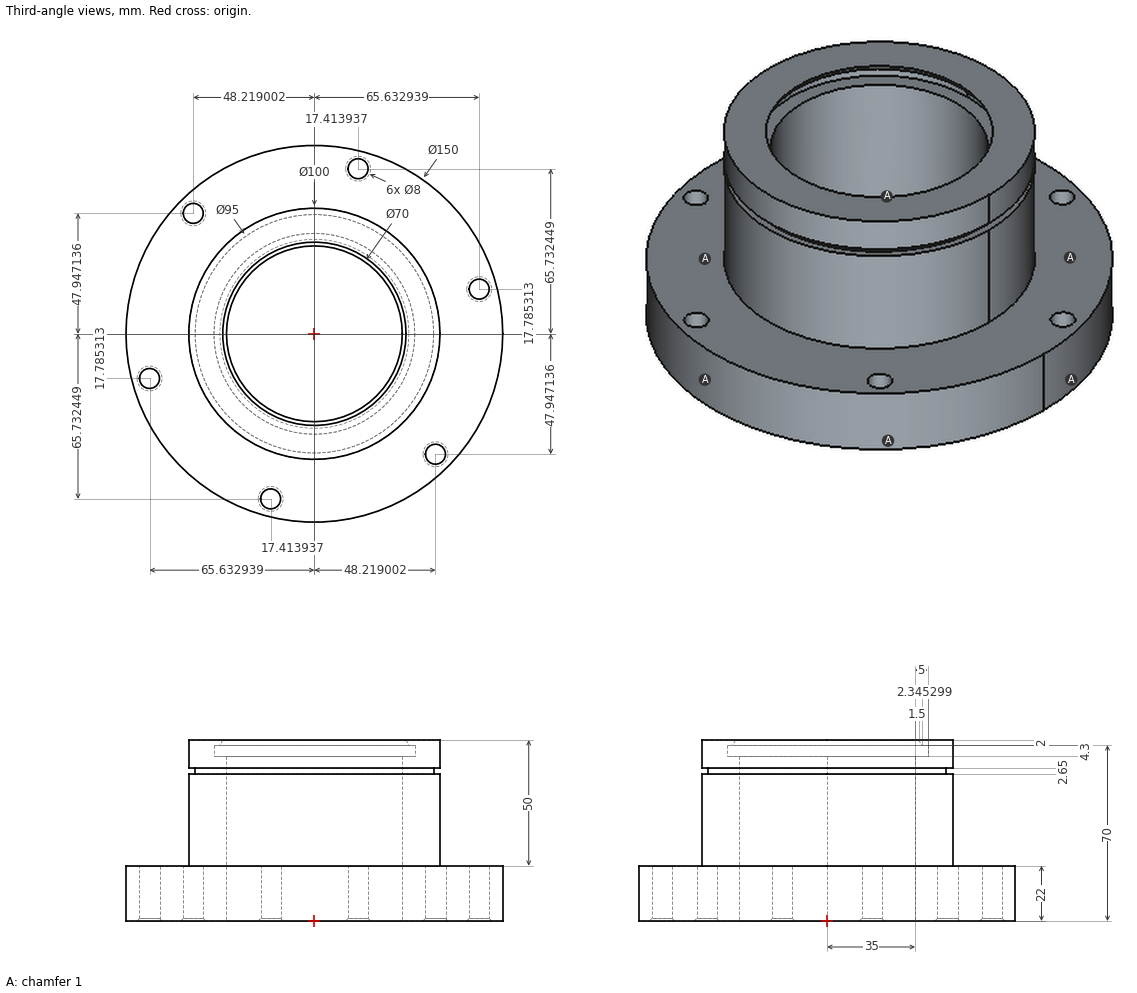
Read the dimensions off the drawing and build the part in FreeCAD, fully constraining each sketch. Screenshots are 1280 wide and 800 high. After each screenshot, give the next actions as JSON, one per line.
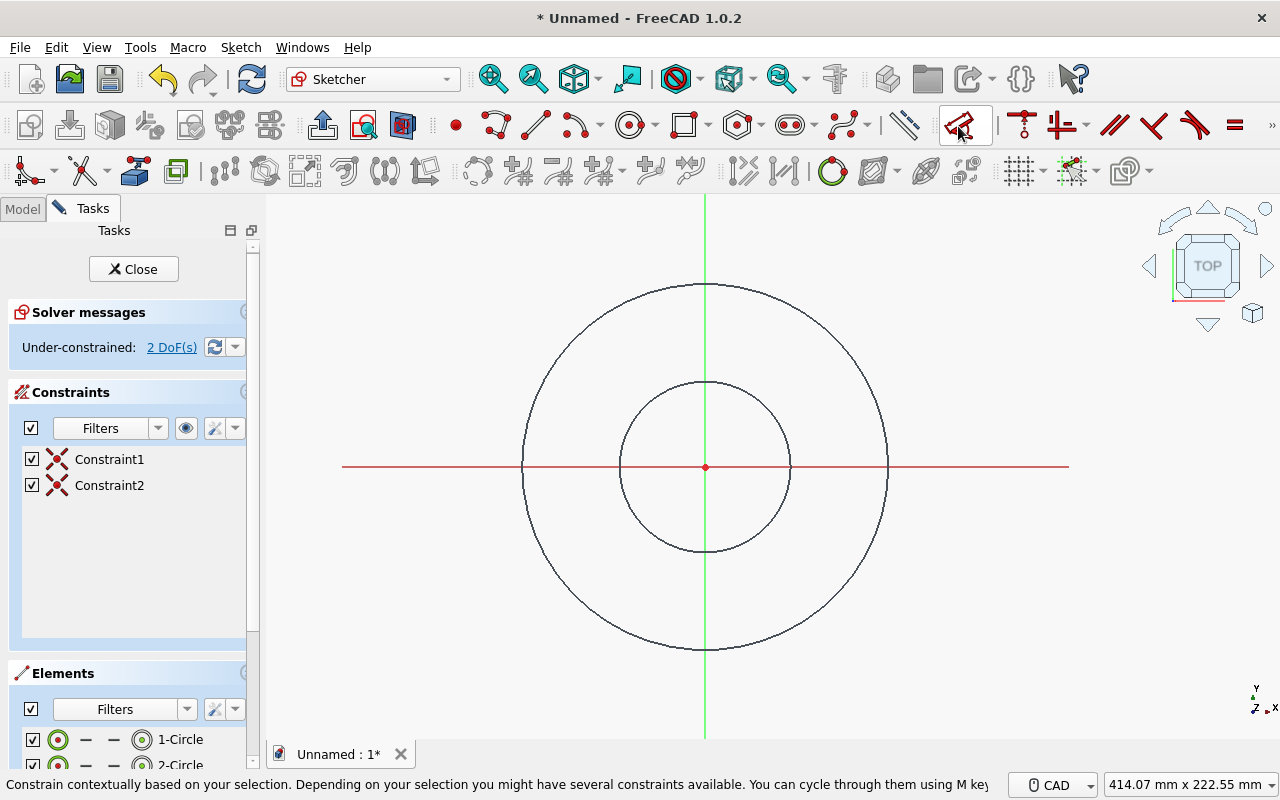
{"action": "left_click", "coordinate": [834, 337]}
{"action": "left_click", "coordinate": [857, 314]}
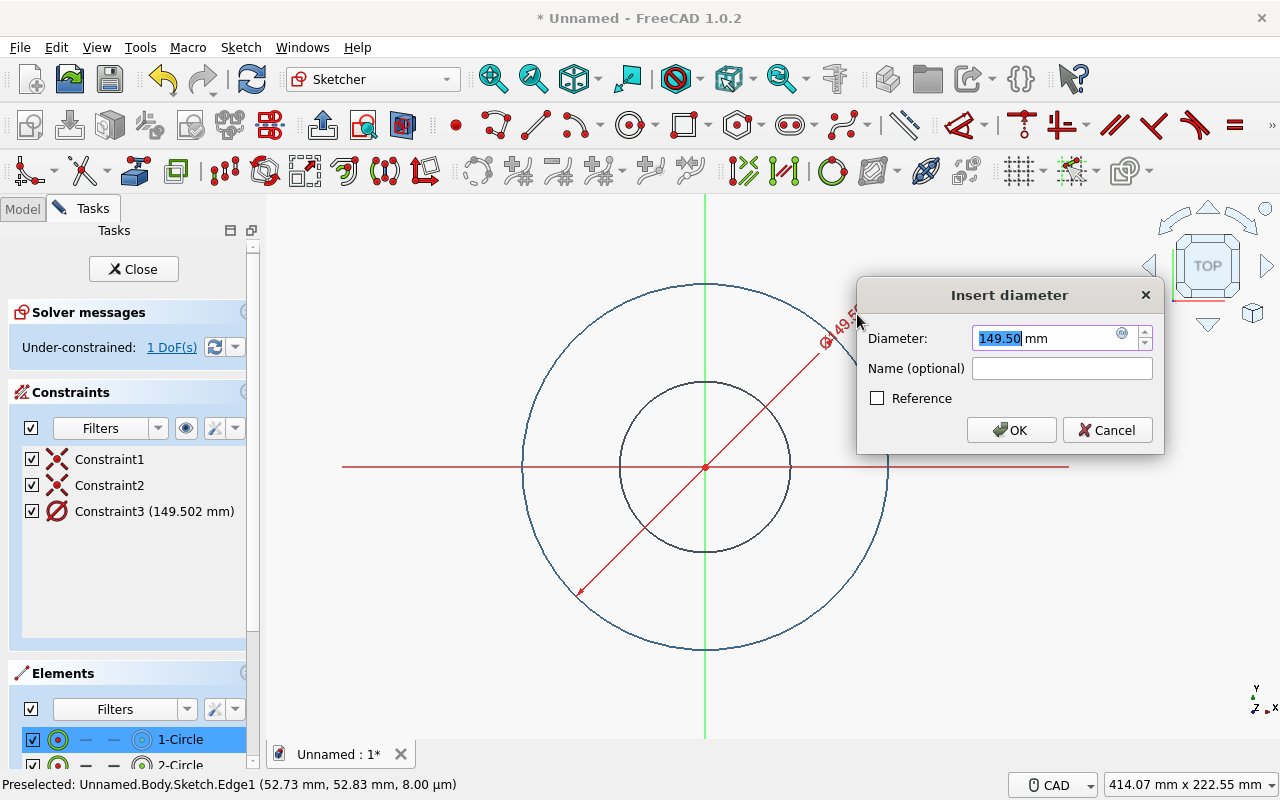
{"action": "type", "text": "150"}
{"action": "key", "text": "Return"}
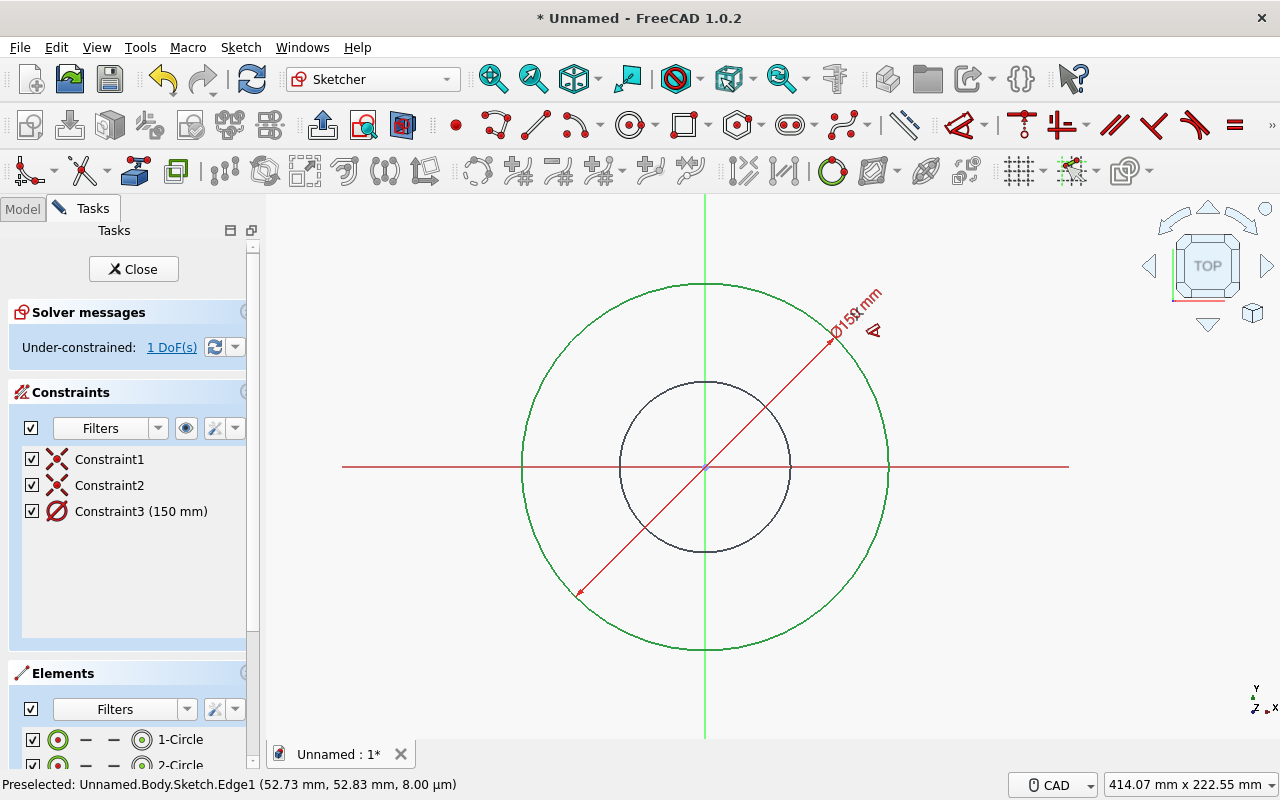
{"action": "left_click", "coordinate": [765, 406]}
{"action": "left_click", "coordinate": [787, 383]}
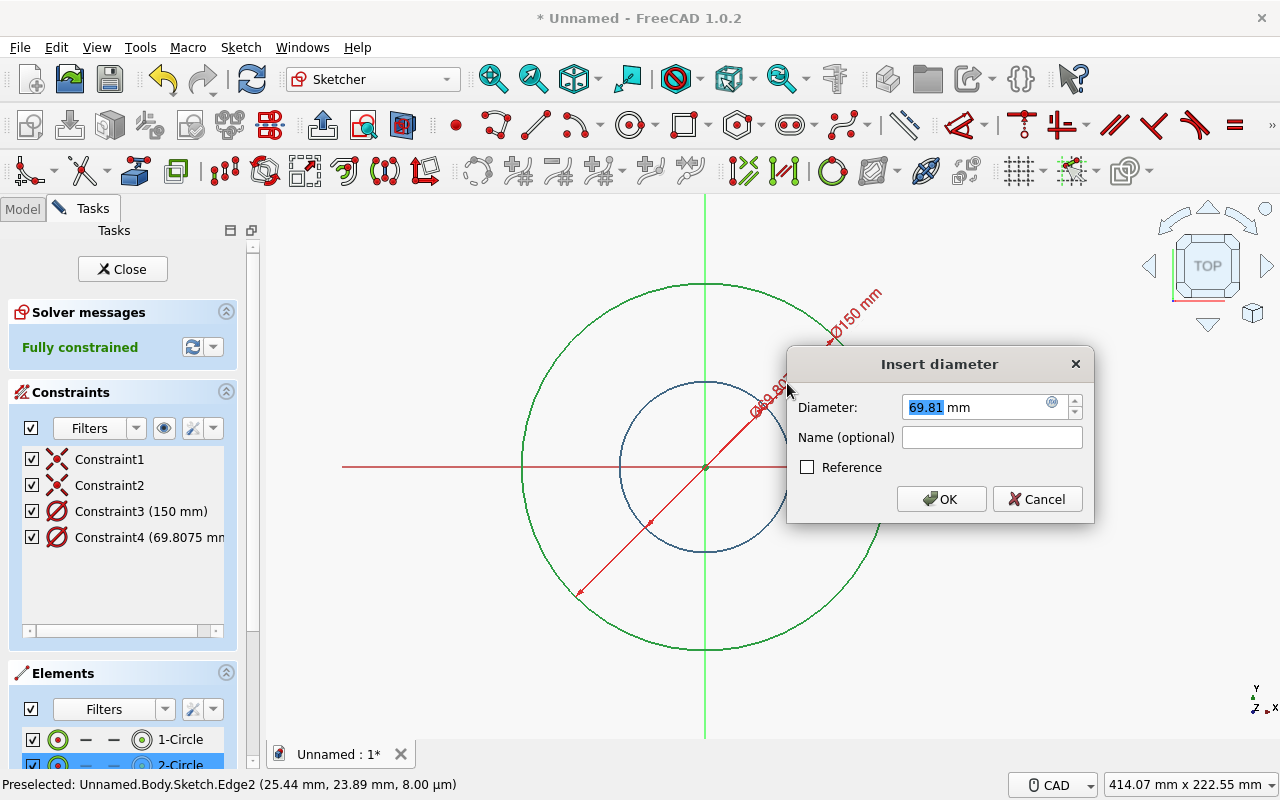
{"action": "type", "text": "70"}
{"action": "key", "text": "Return"}
{"action": "key", "text": "Escape"}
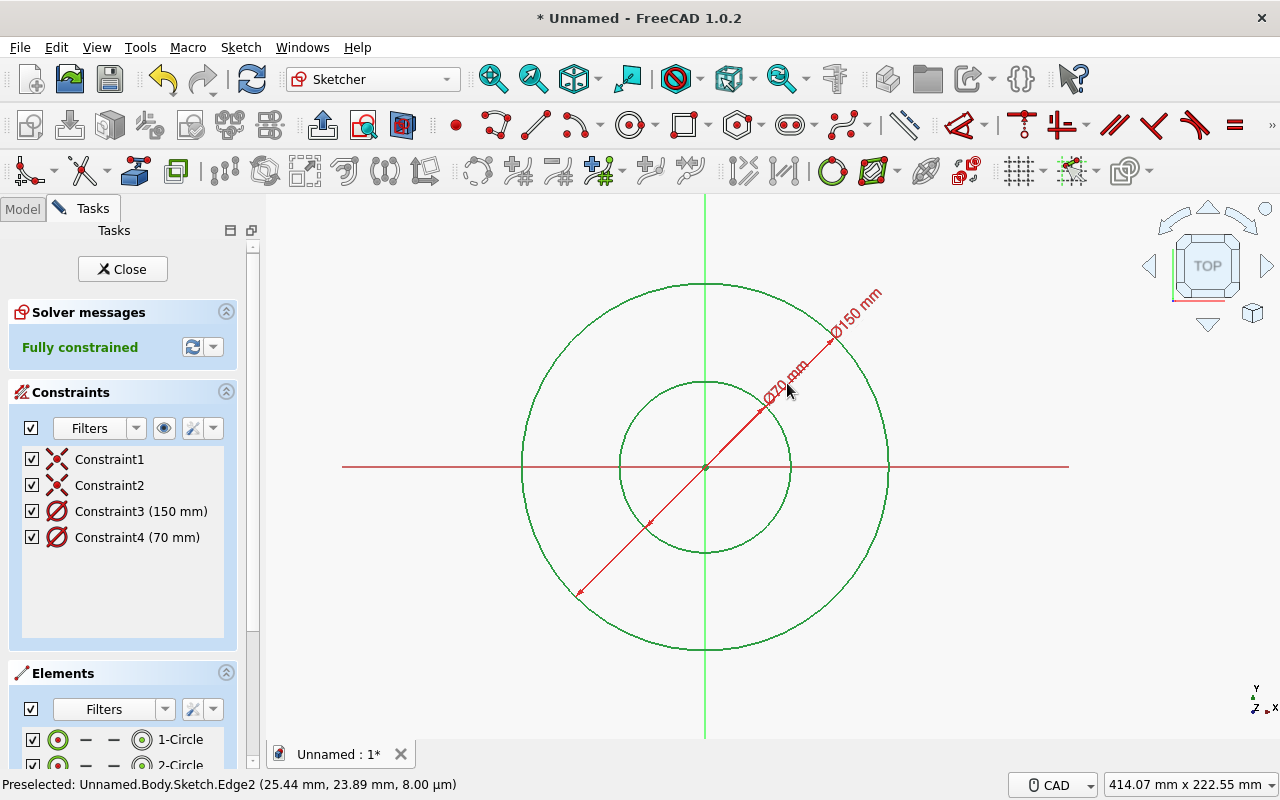
{"action": "left_click", "coordinate": [123, 269]}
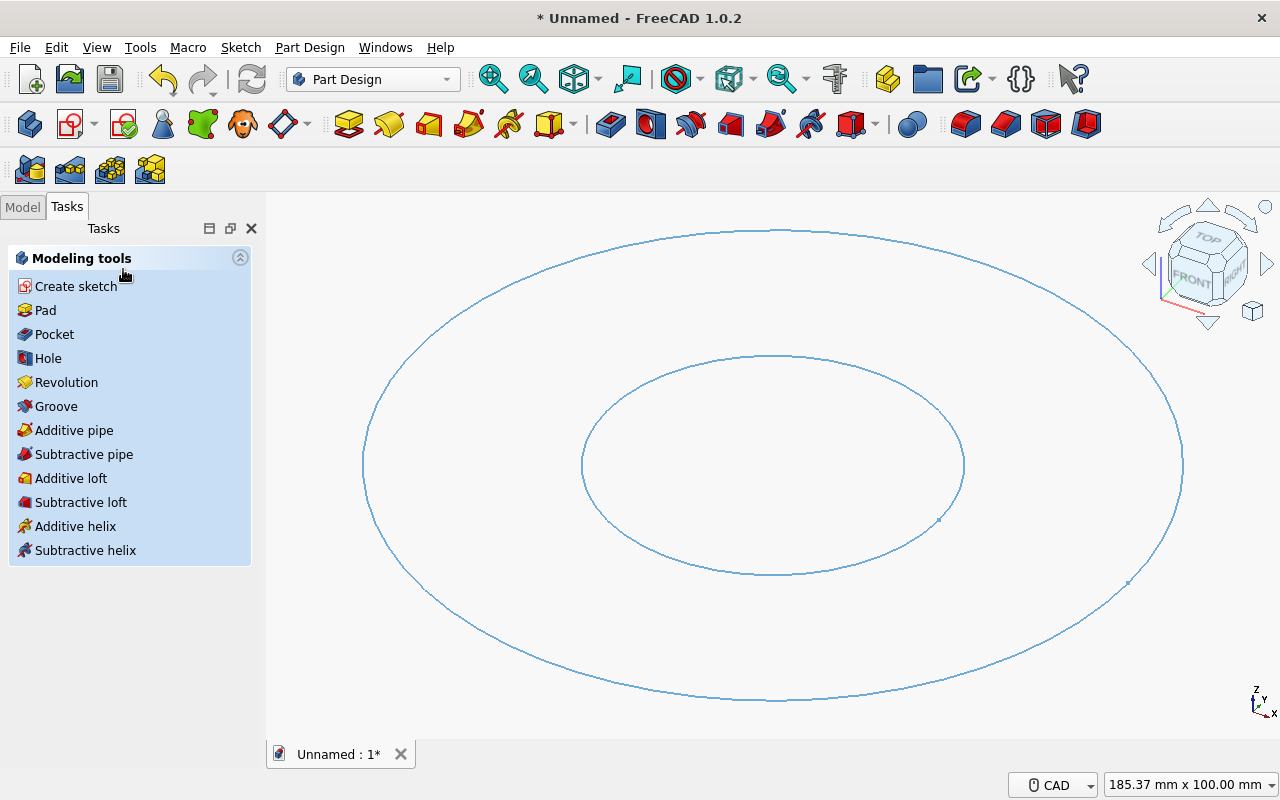
{"action": "left_click", "coordinate": [350, 124]}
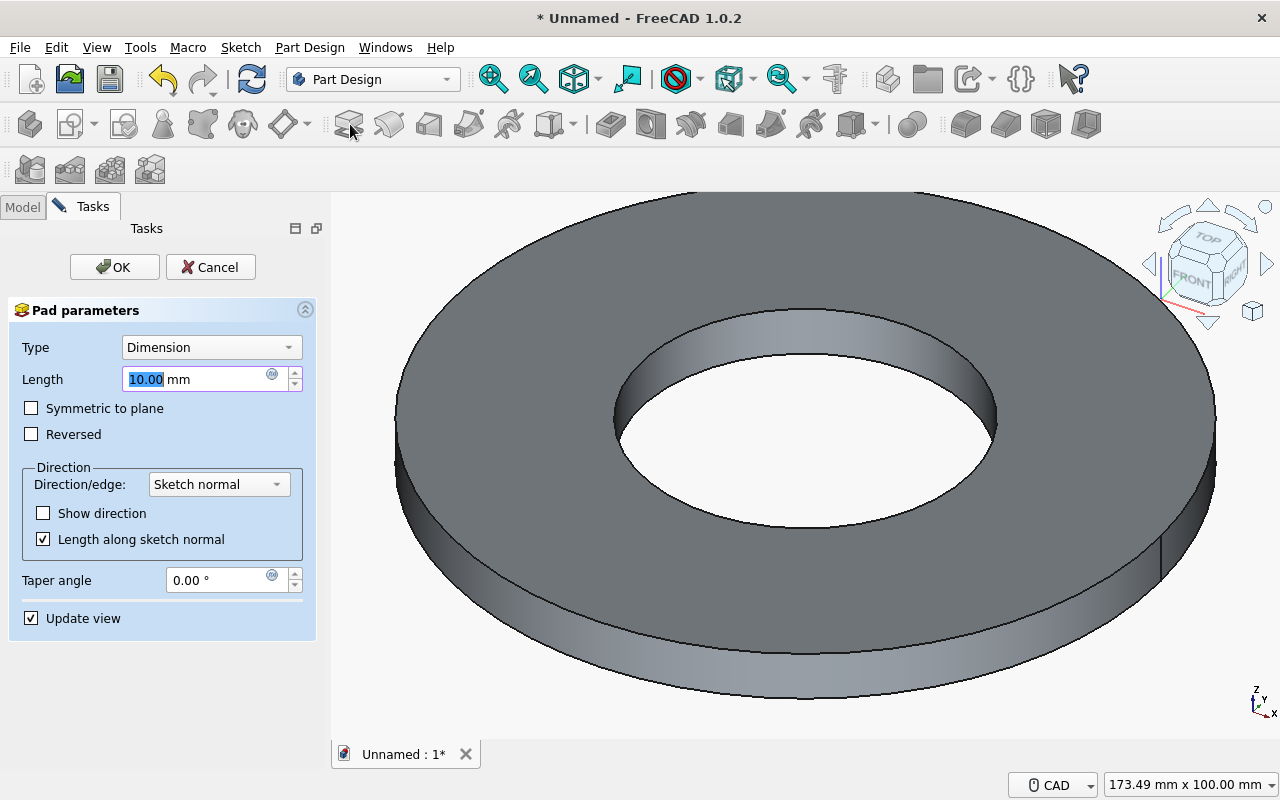
{"action": "type", "text": "22"}
{"action": "key", "text": "Tab"}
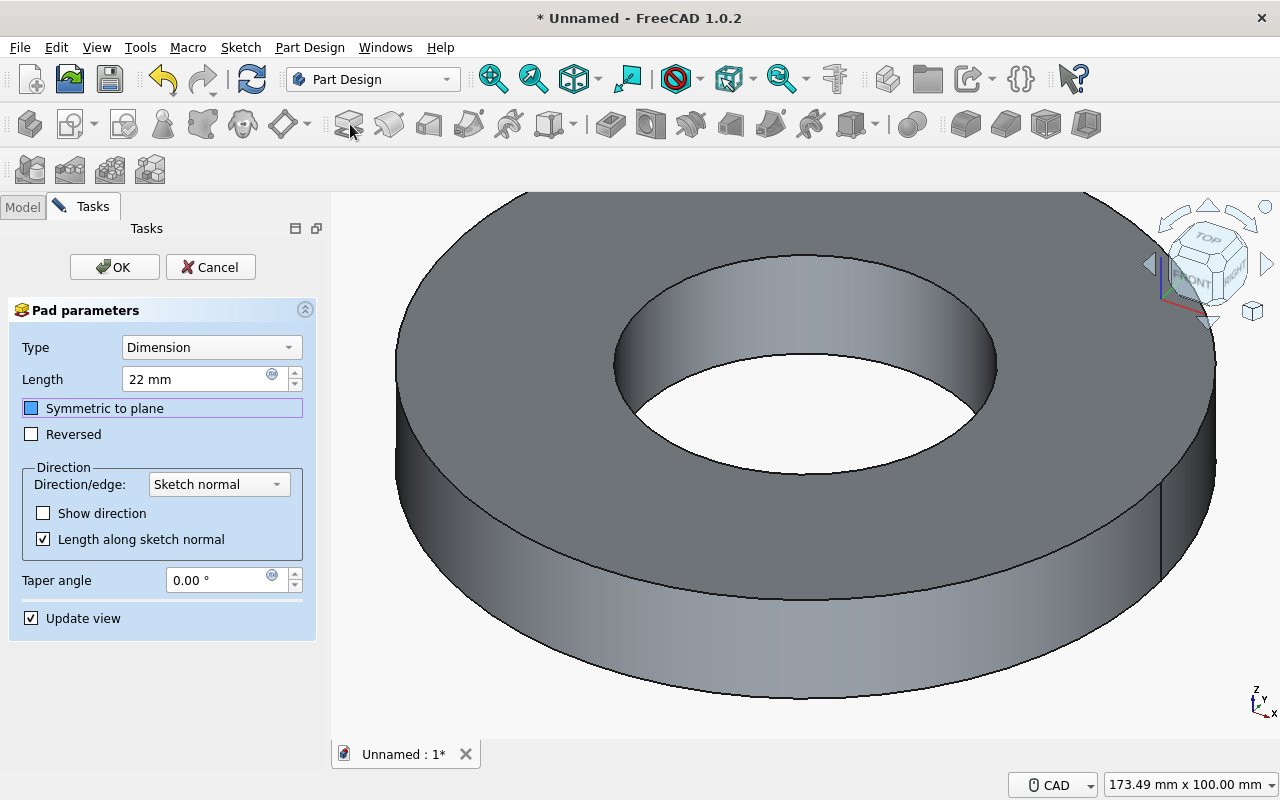
{"action": "left_click", "coordinate": [115, 267]}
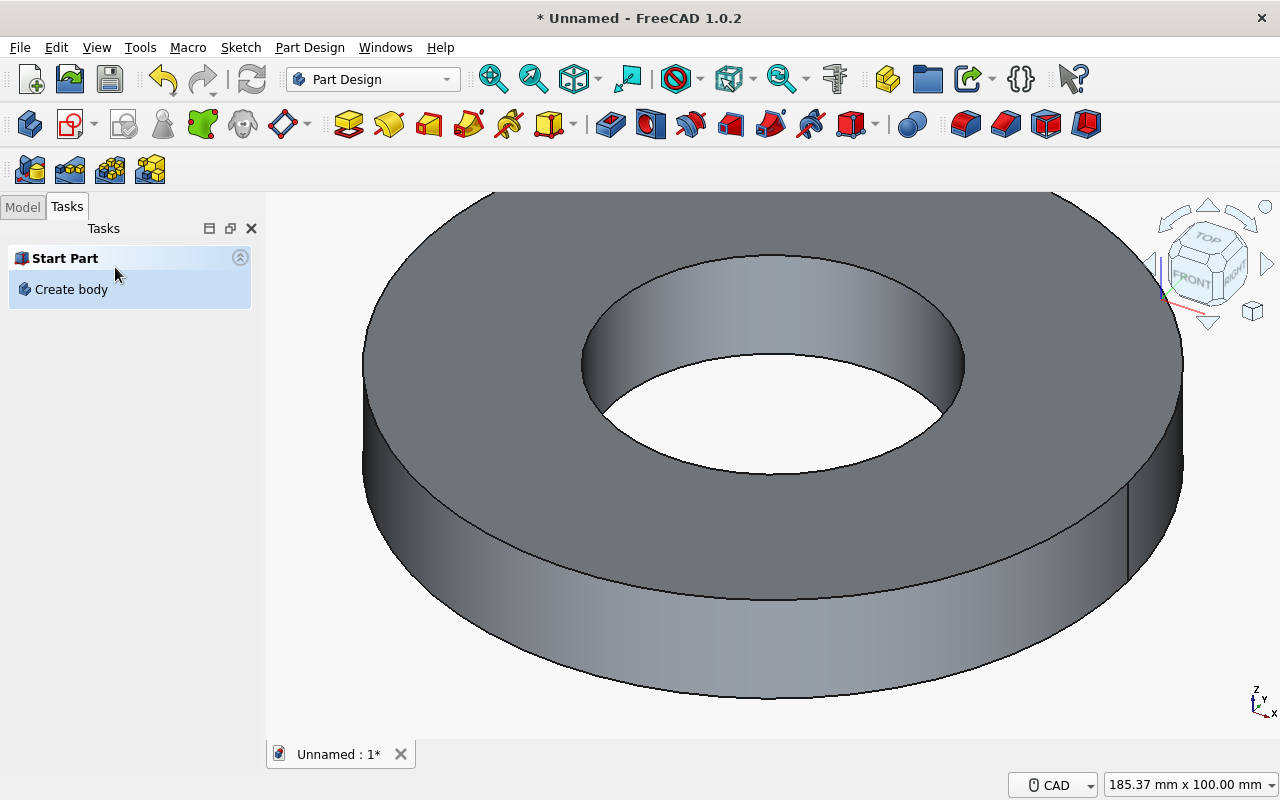
{"action": "left_click", "coordinate": [494, 80]}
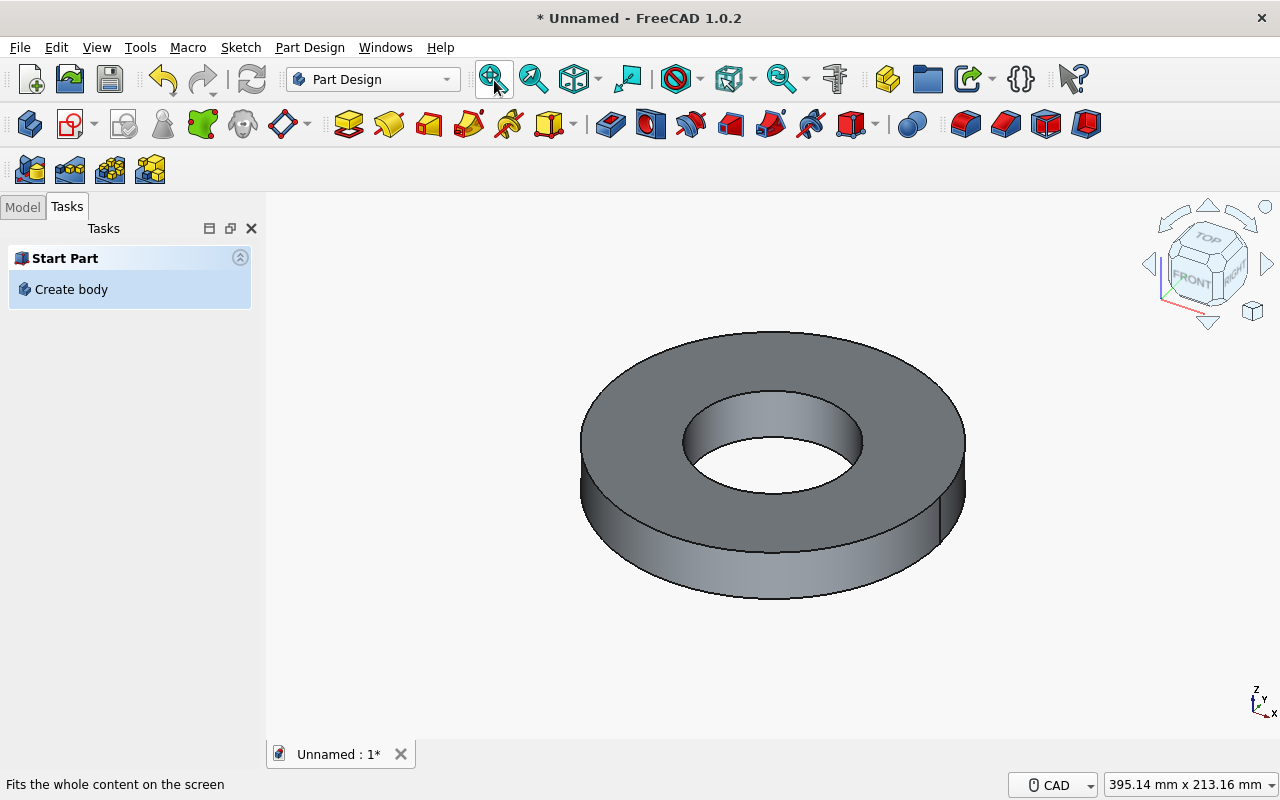
{"action": "left_click", "coordinate": [813, 528]}